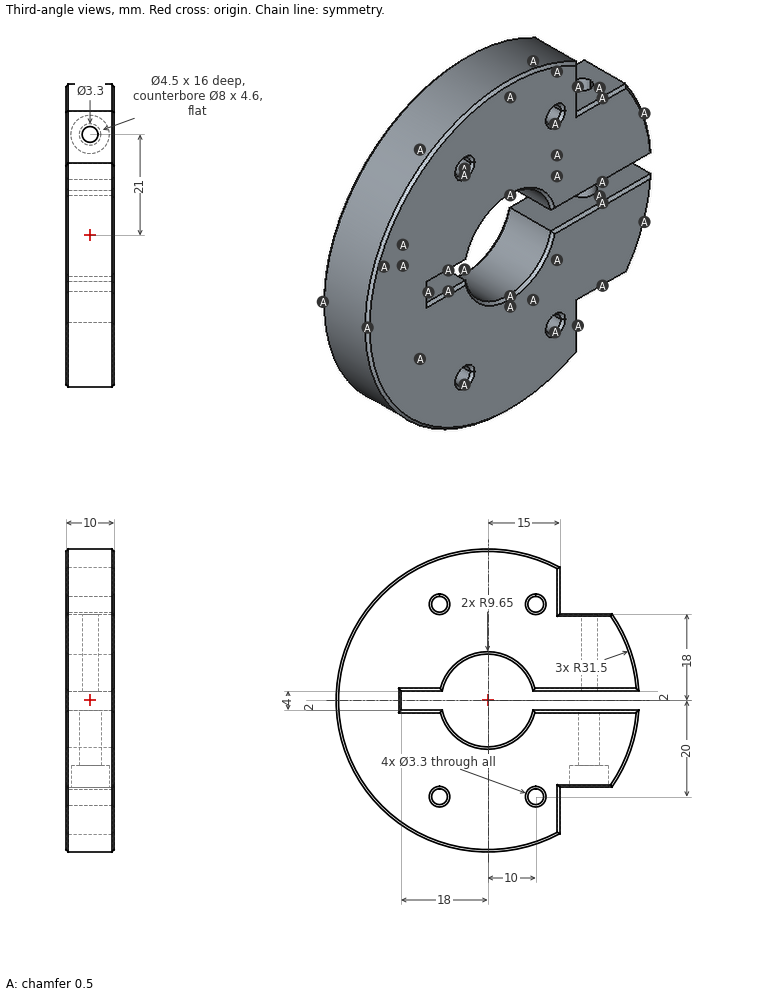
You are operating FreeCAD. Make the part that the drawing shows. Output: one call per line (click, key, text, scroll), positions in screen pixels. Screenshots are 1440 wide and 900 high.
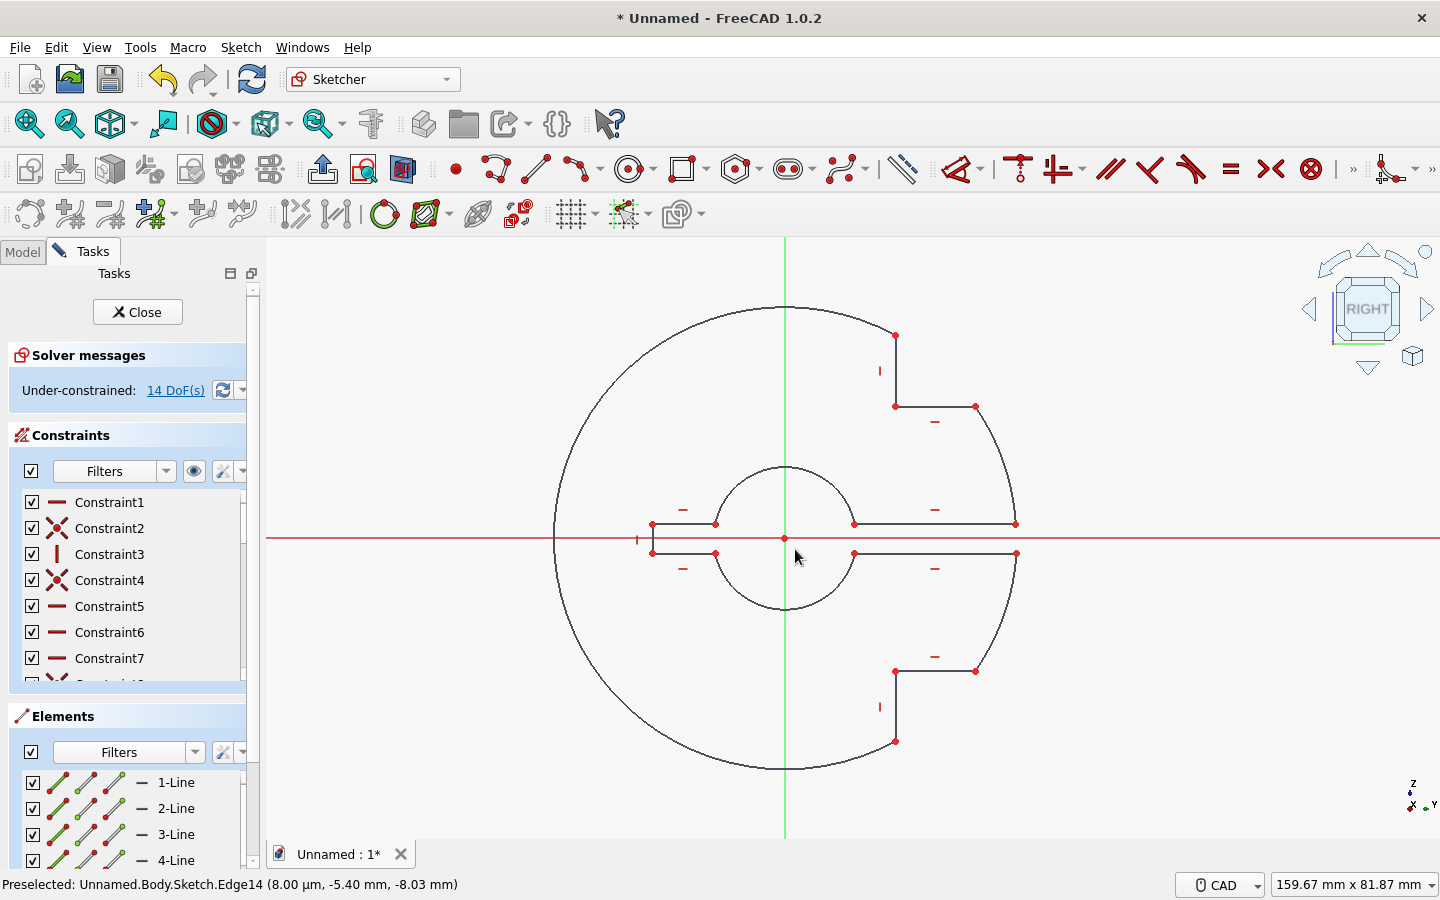
click(1010, 487)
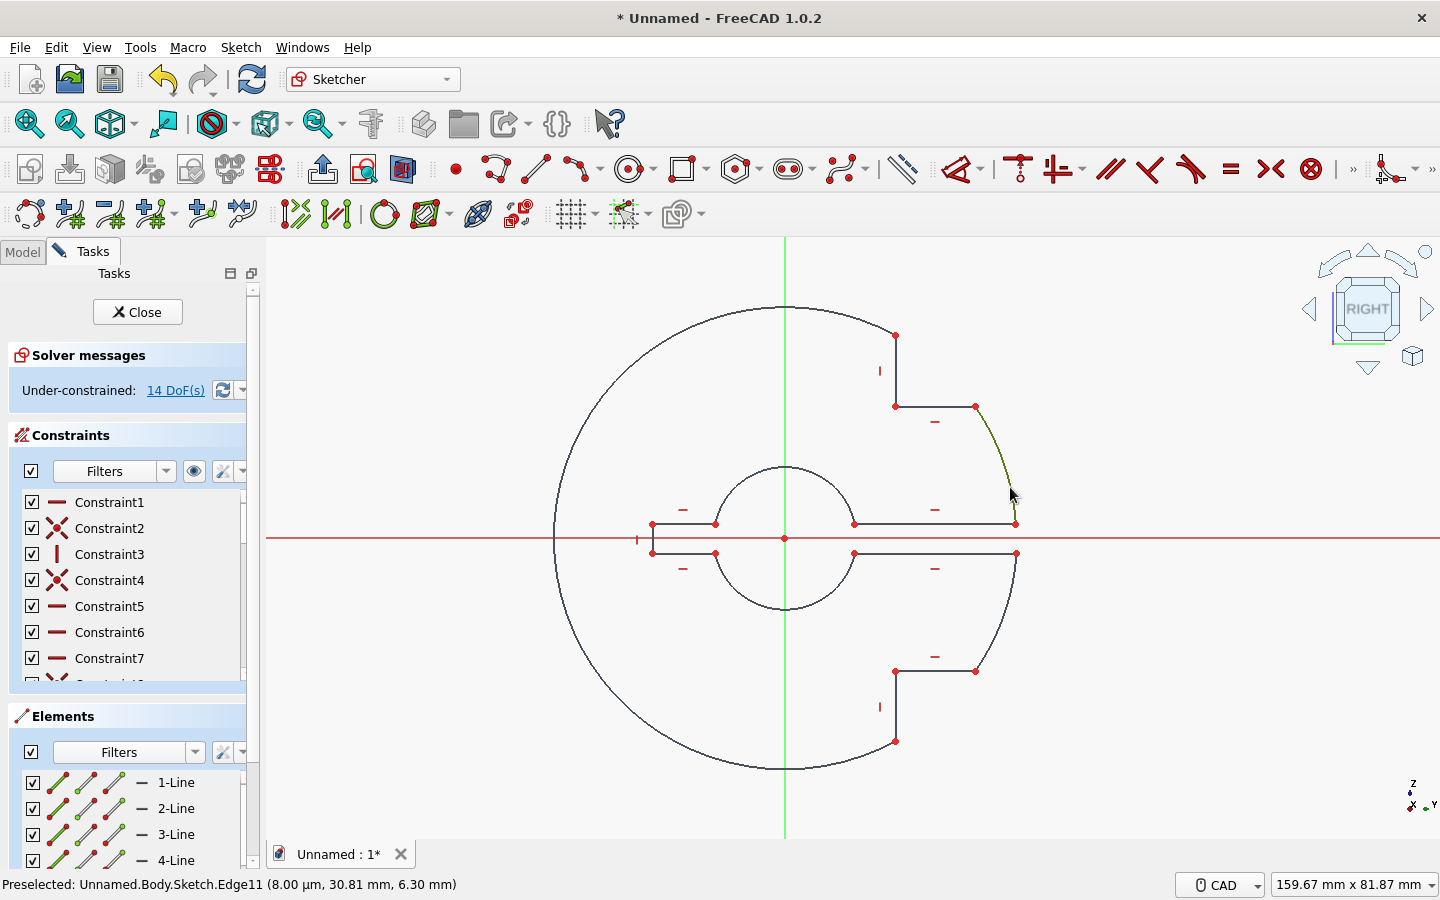
click(629, 368)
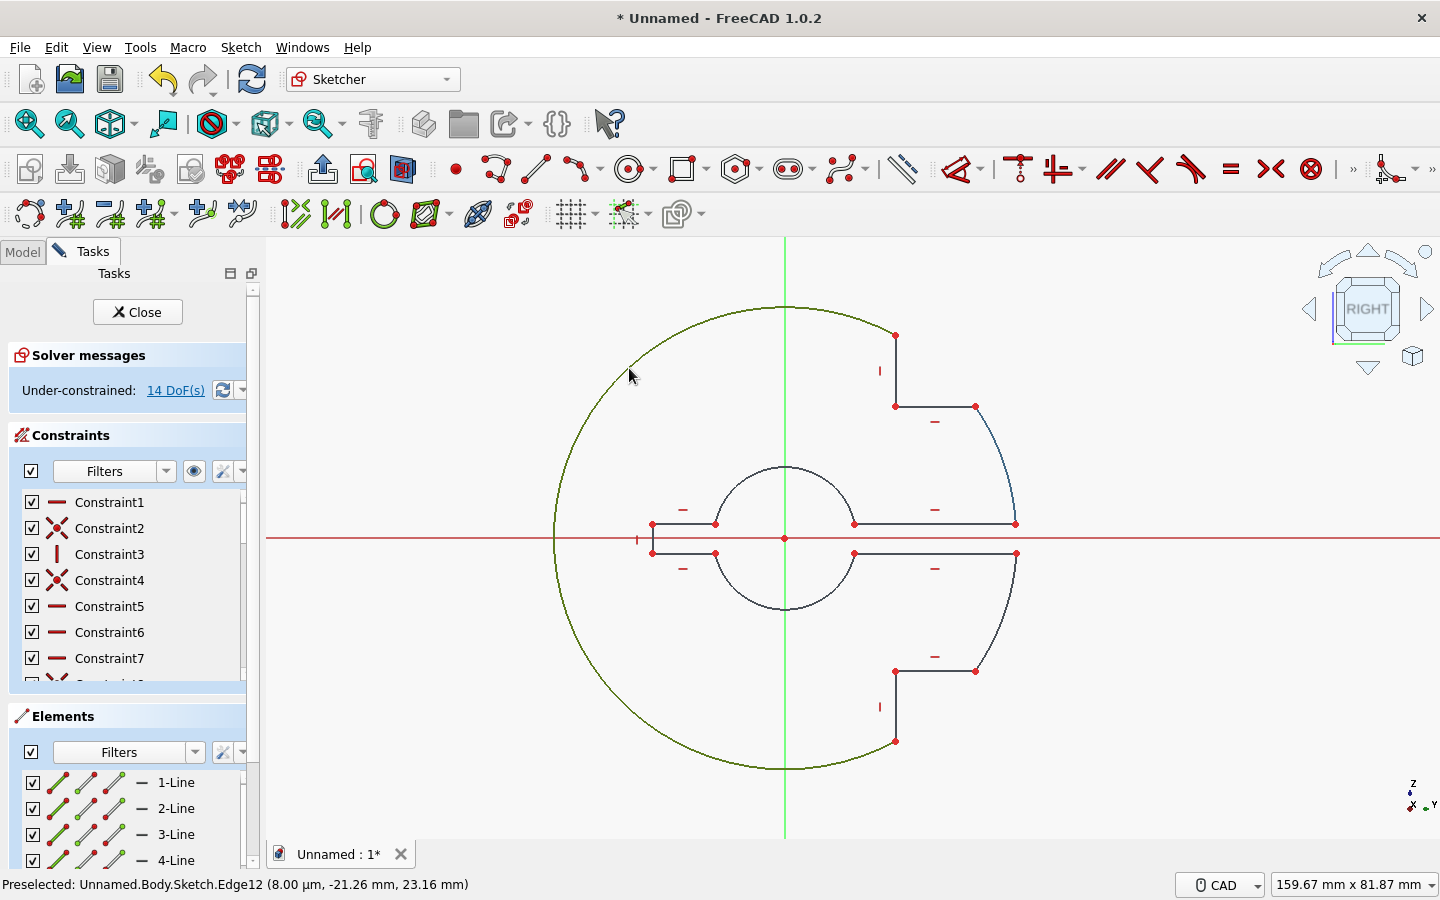
click(994, 639)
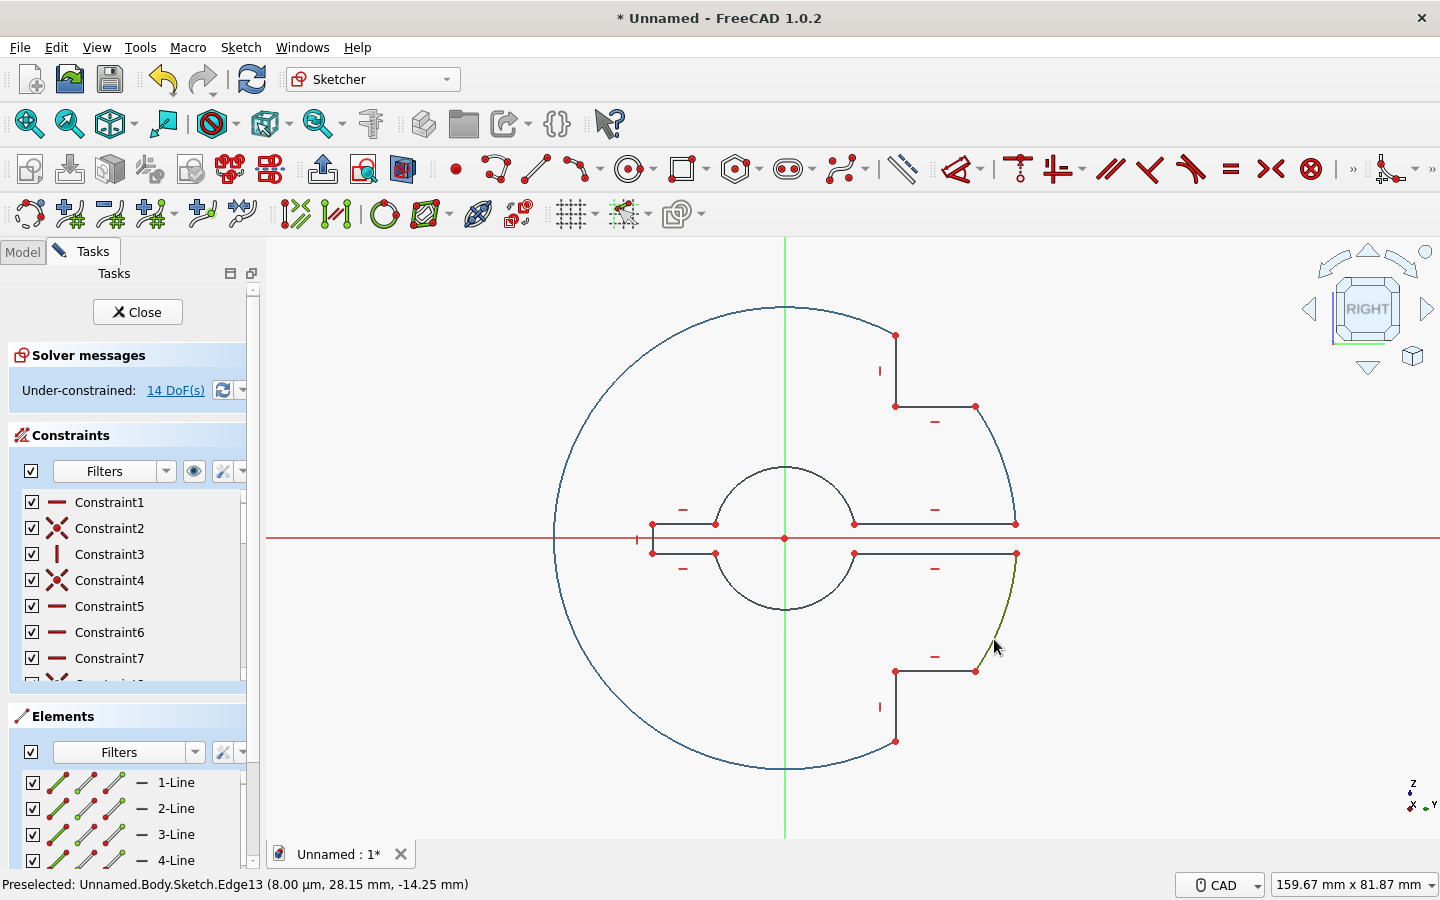
key(e)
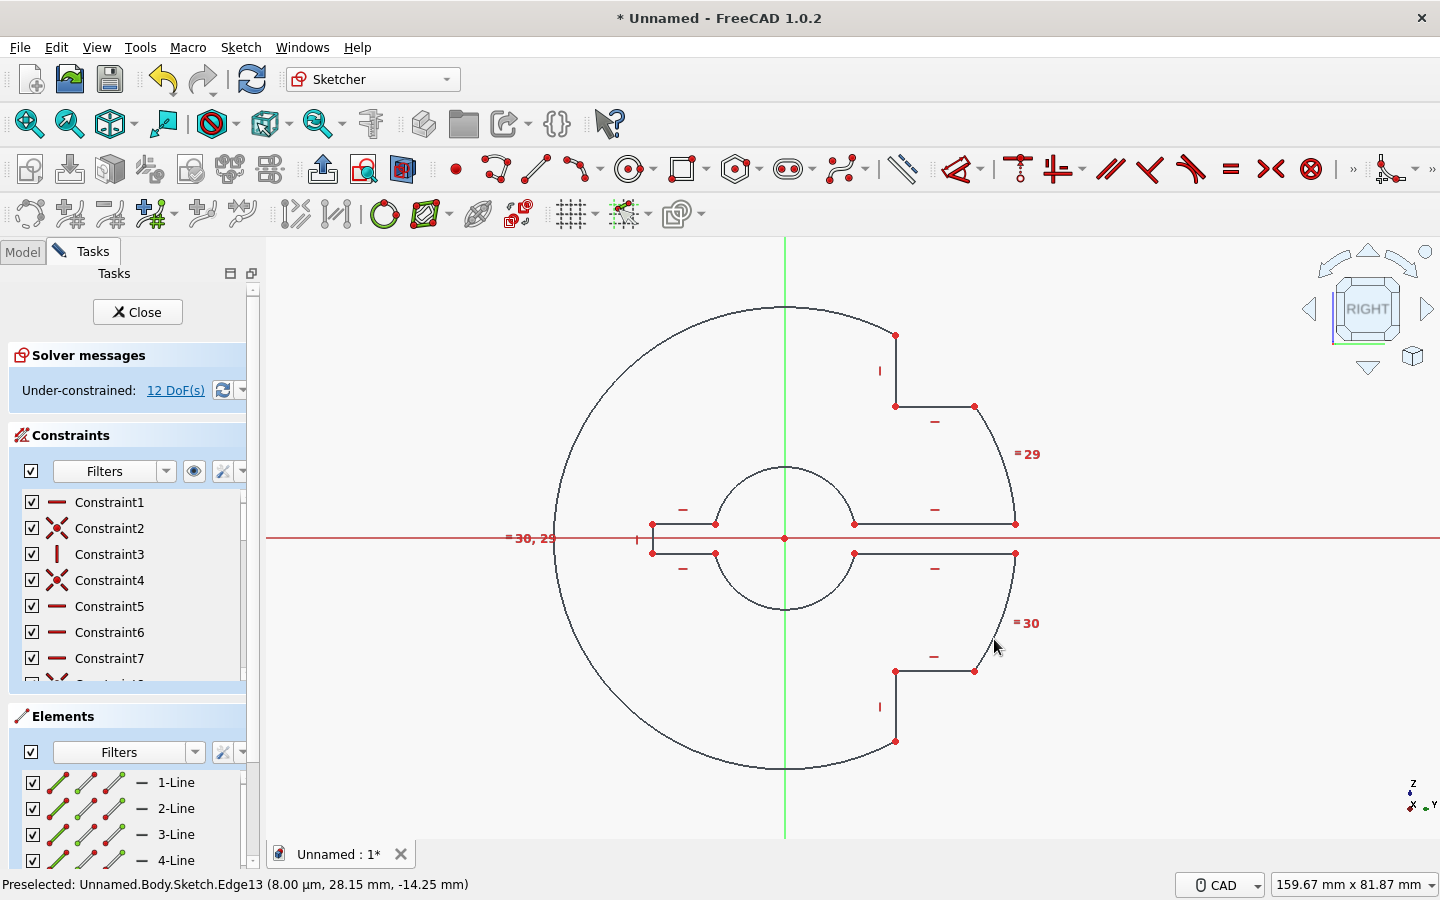
click(822, 478)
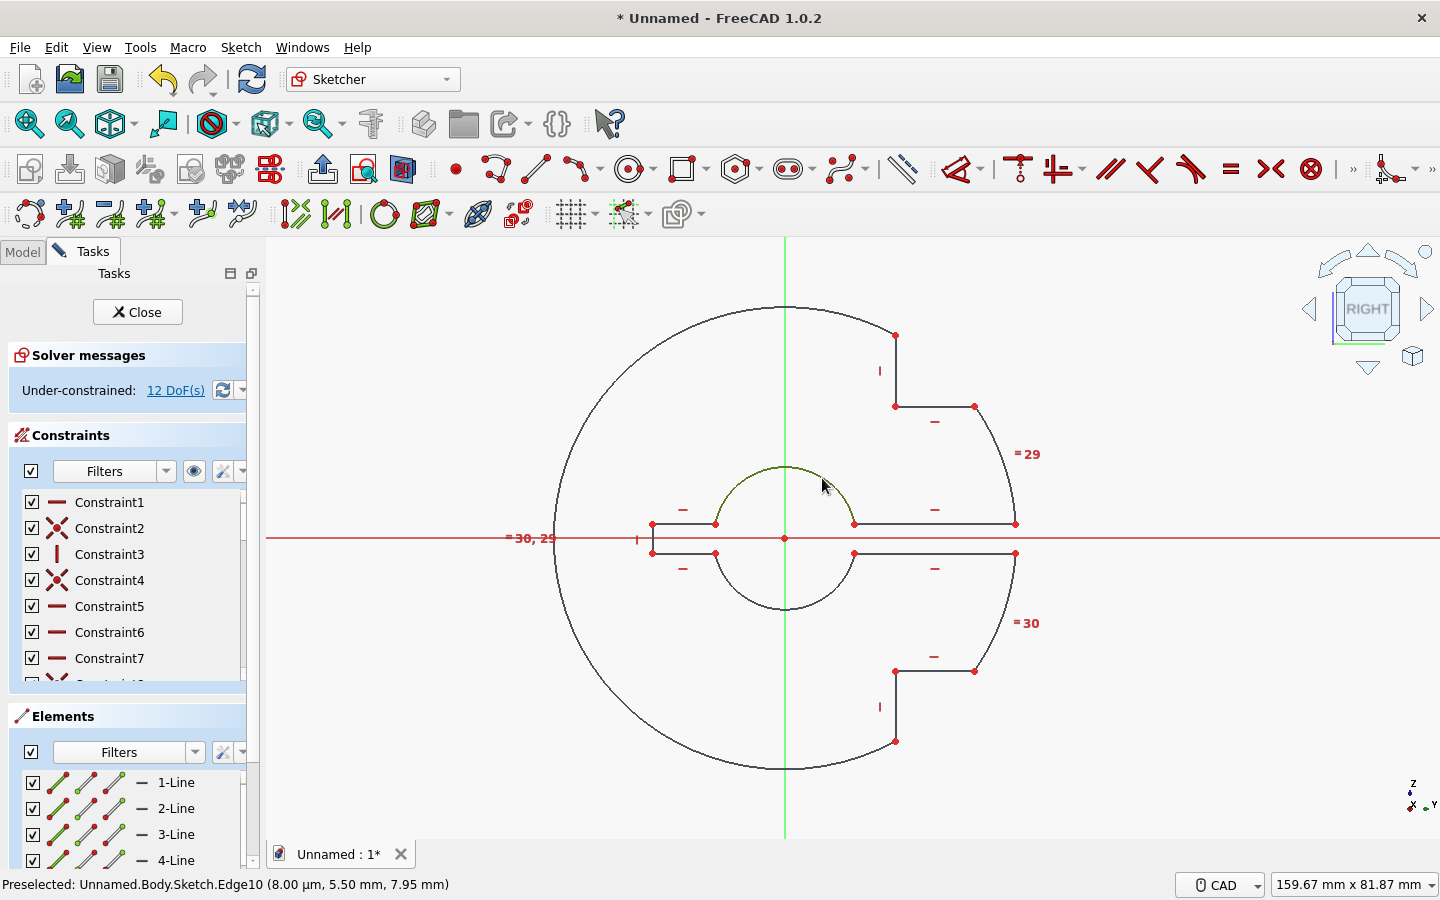
click(748, 600)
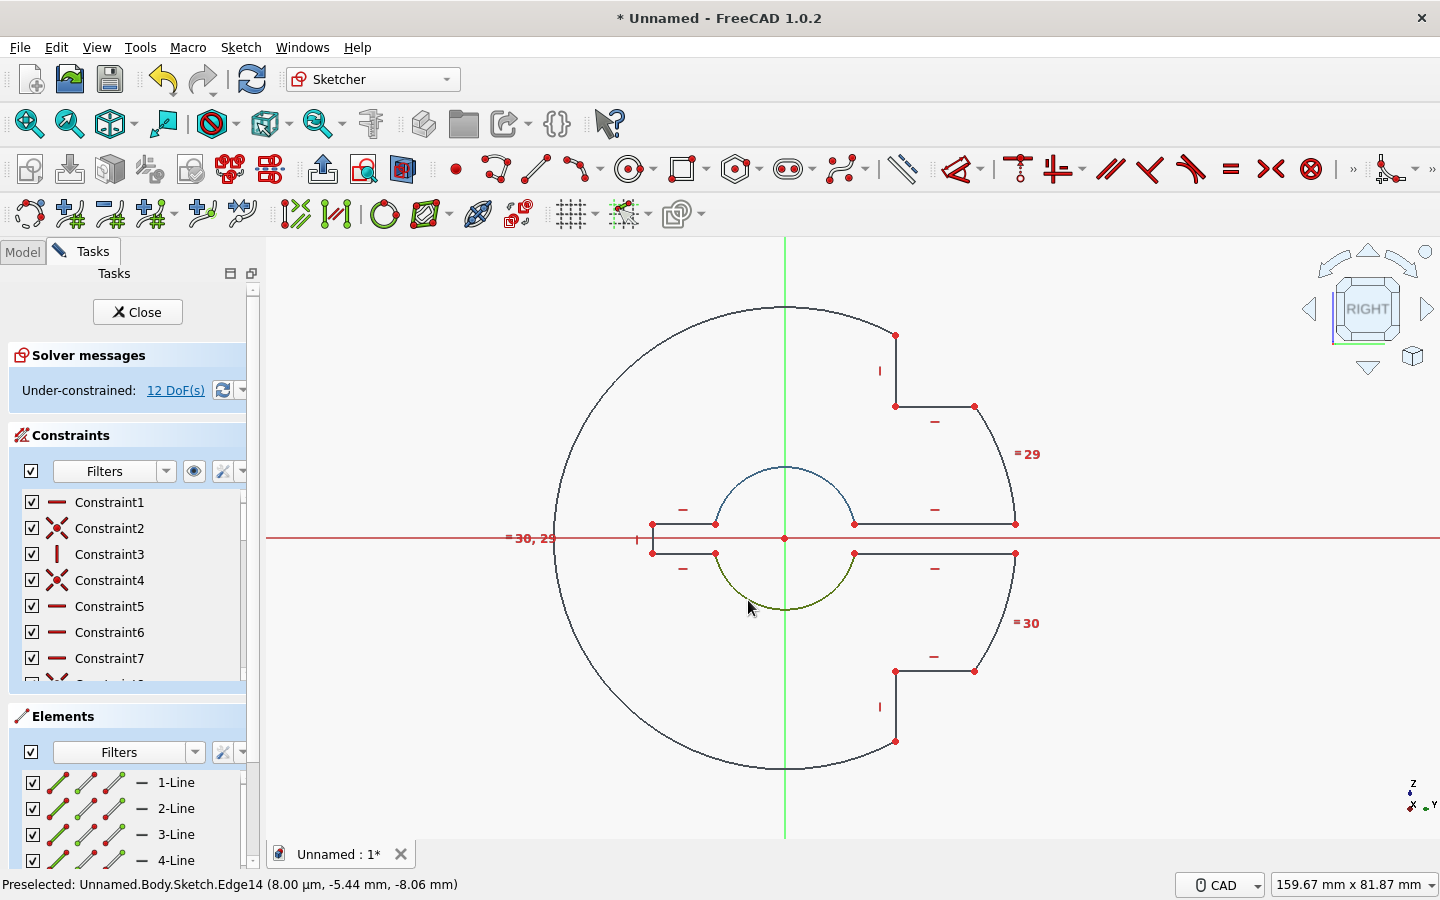
key(e)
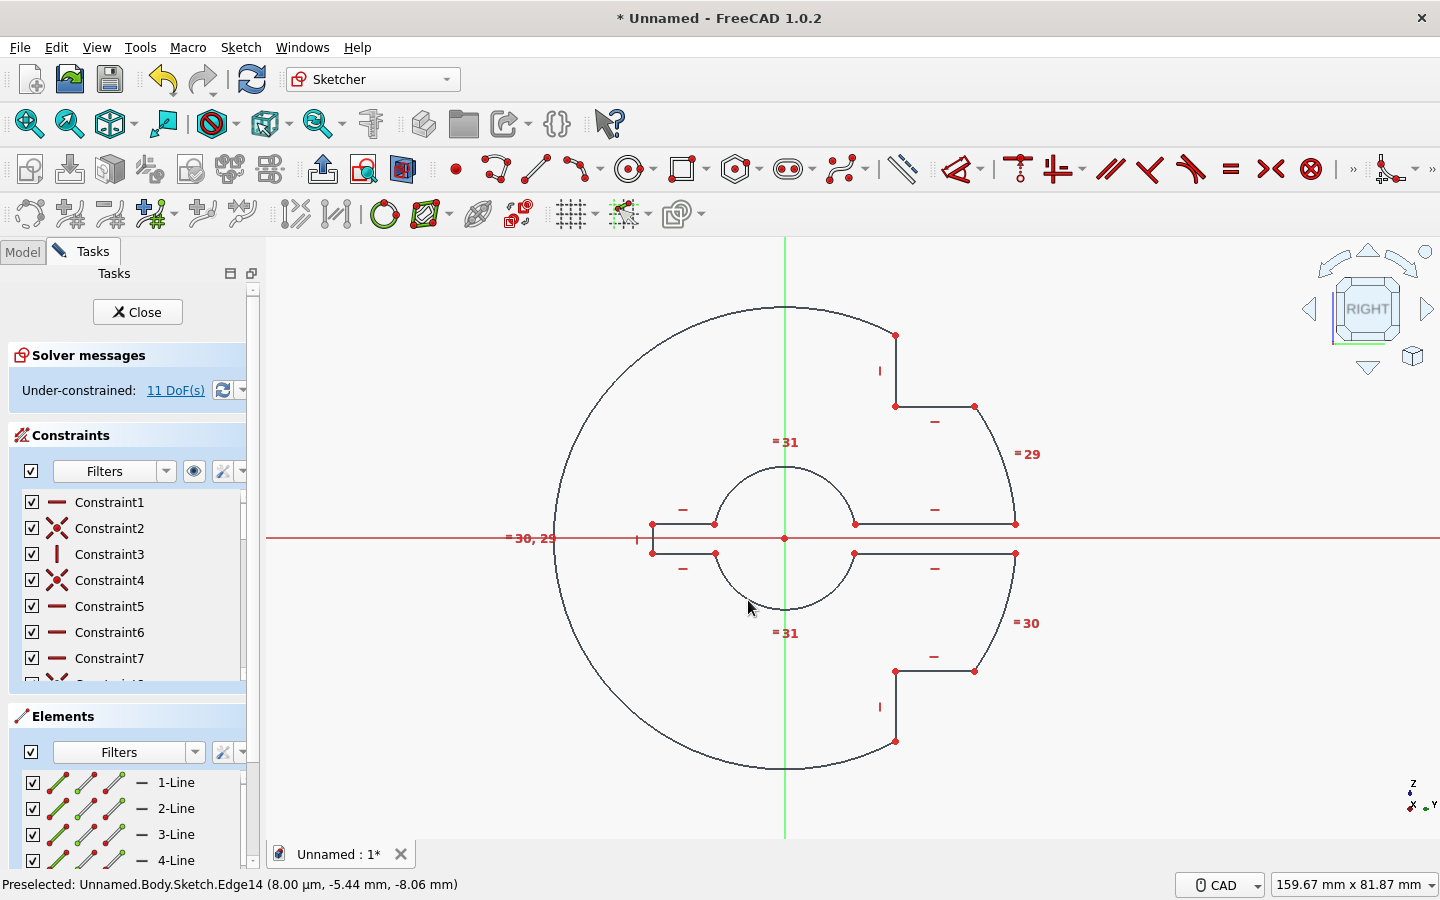
click(896, 407)